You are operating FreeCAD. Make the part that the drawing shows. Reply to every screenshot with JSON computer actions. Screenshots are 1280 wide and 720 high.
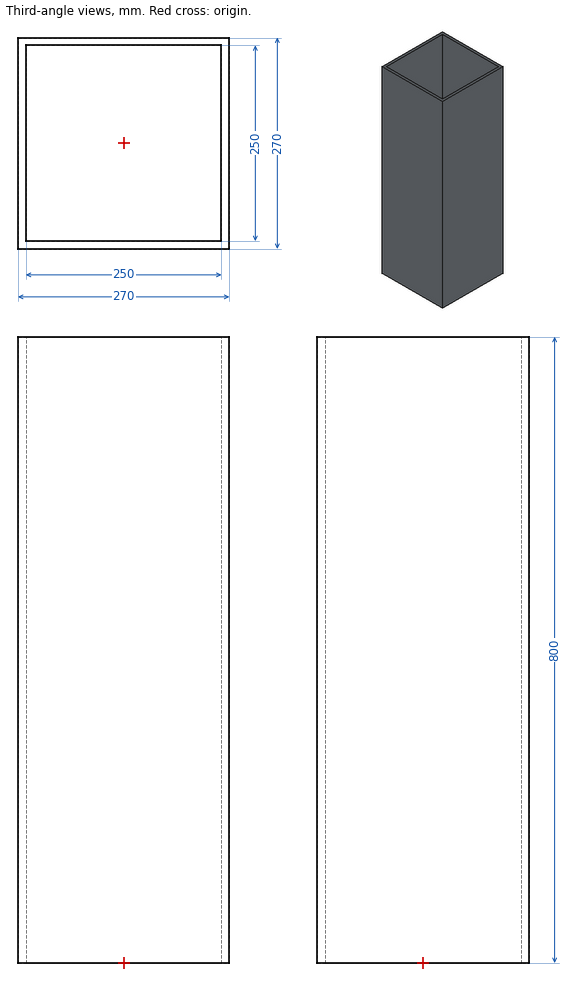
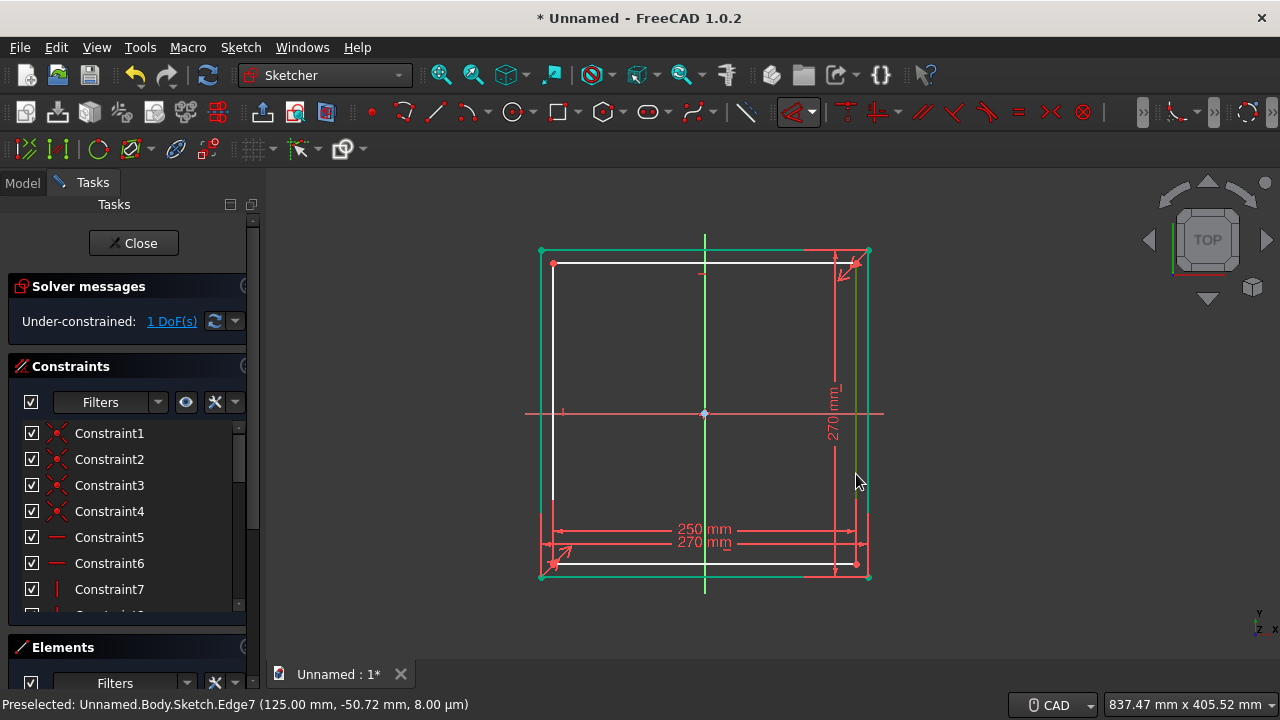
{"action": "left_click", "coordinate": [814, 112]}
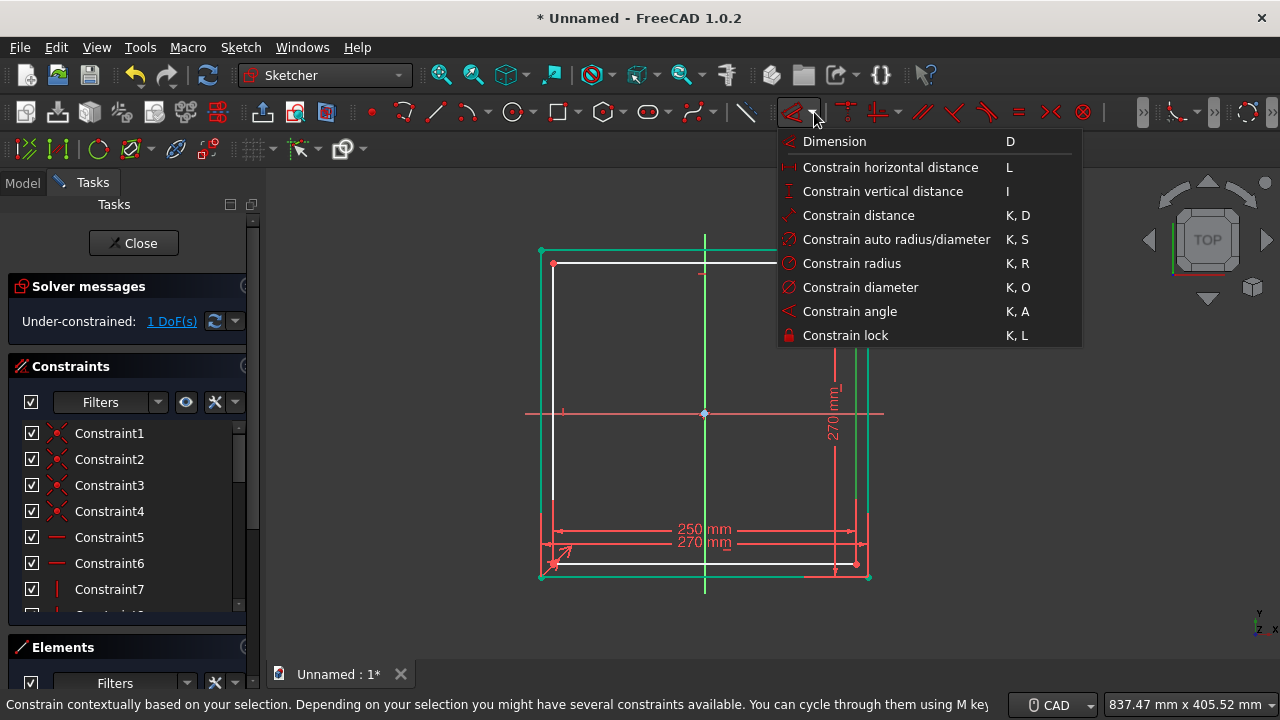
{"action": "left_click", "coordinate": [930, 191]}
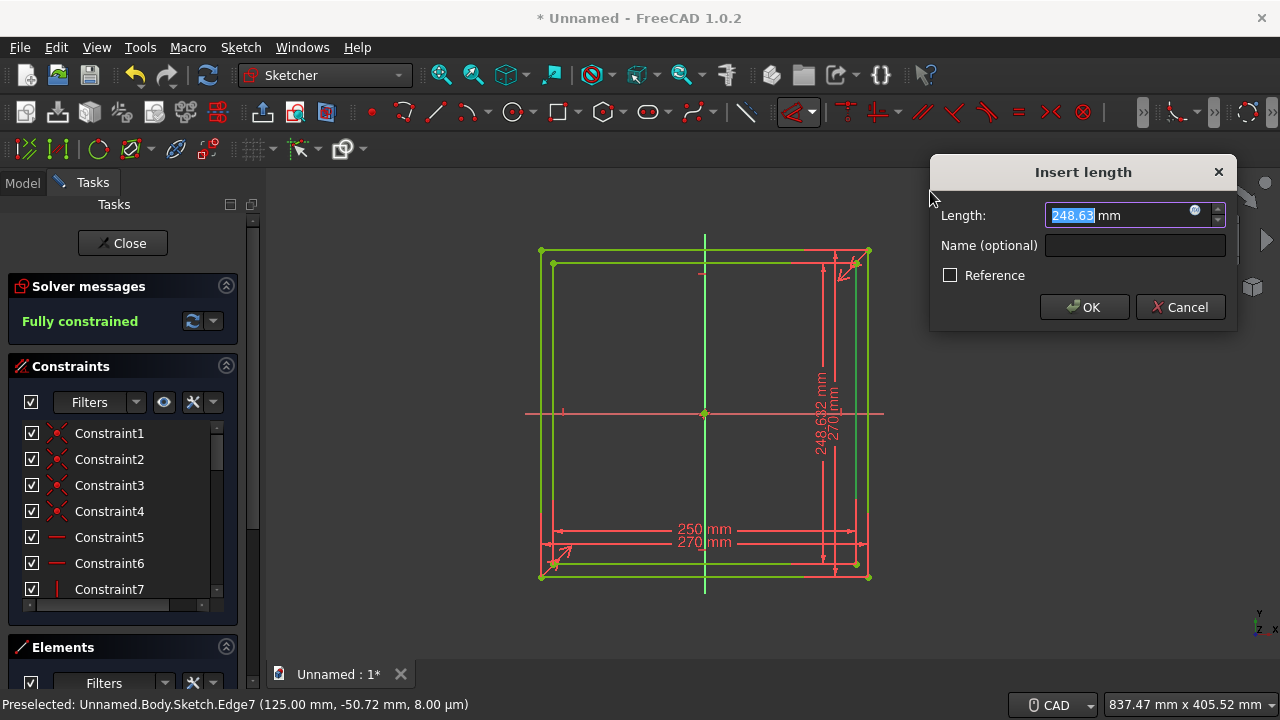
{"action": "type", "text": "250"}
{"action": "key", "text": "Return"}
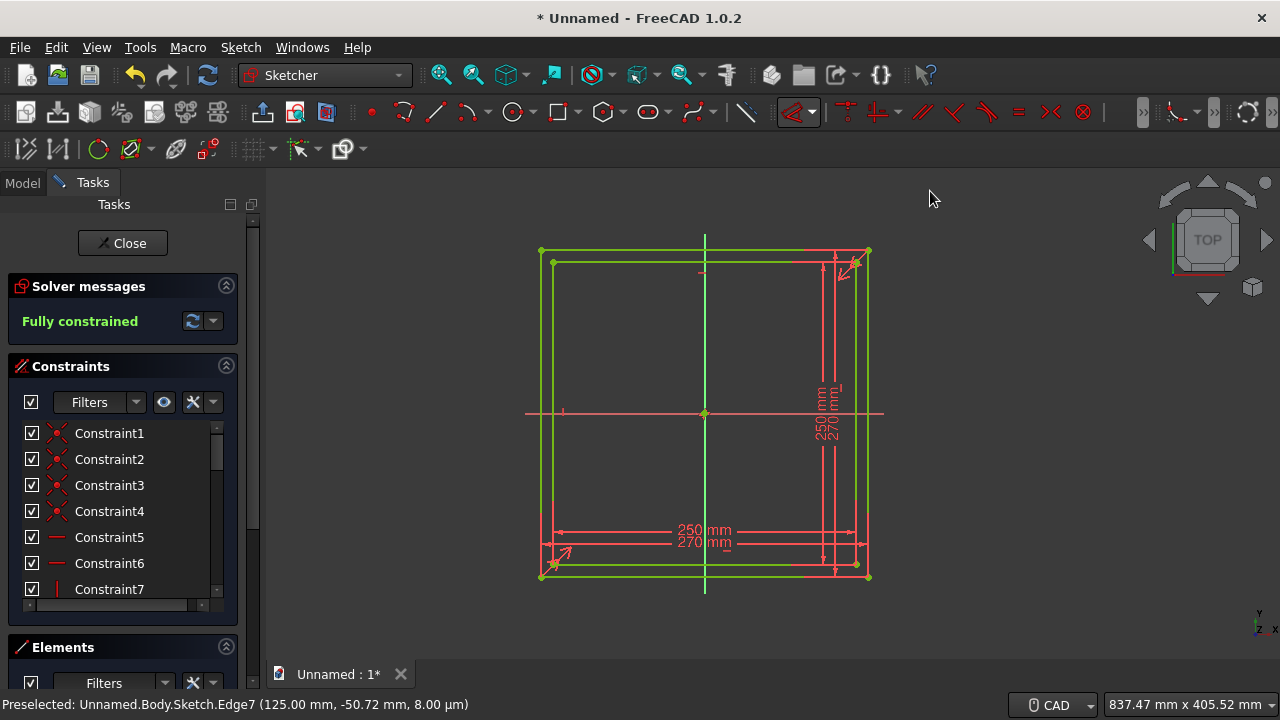
{"action": "left_click", "coordinate": [123, 243]}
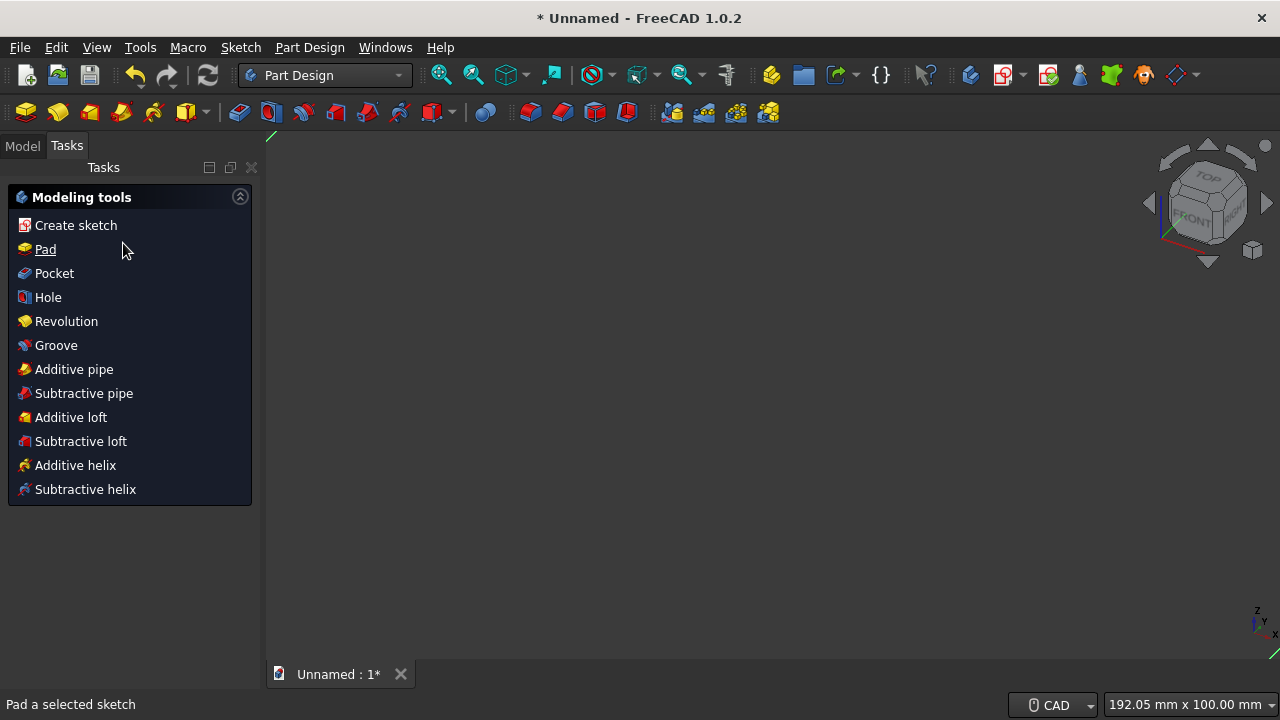
{"action": "left_click", "coordinate": [26, 112]}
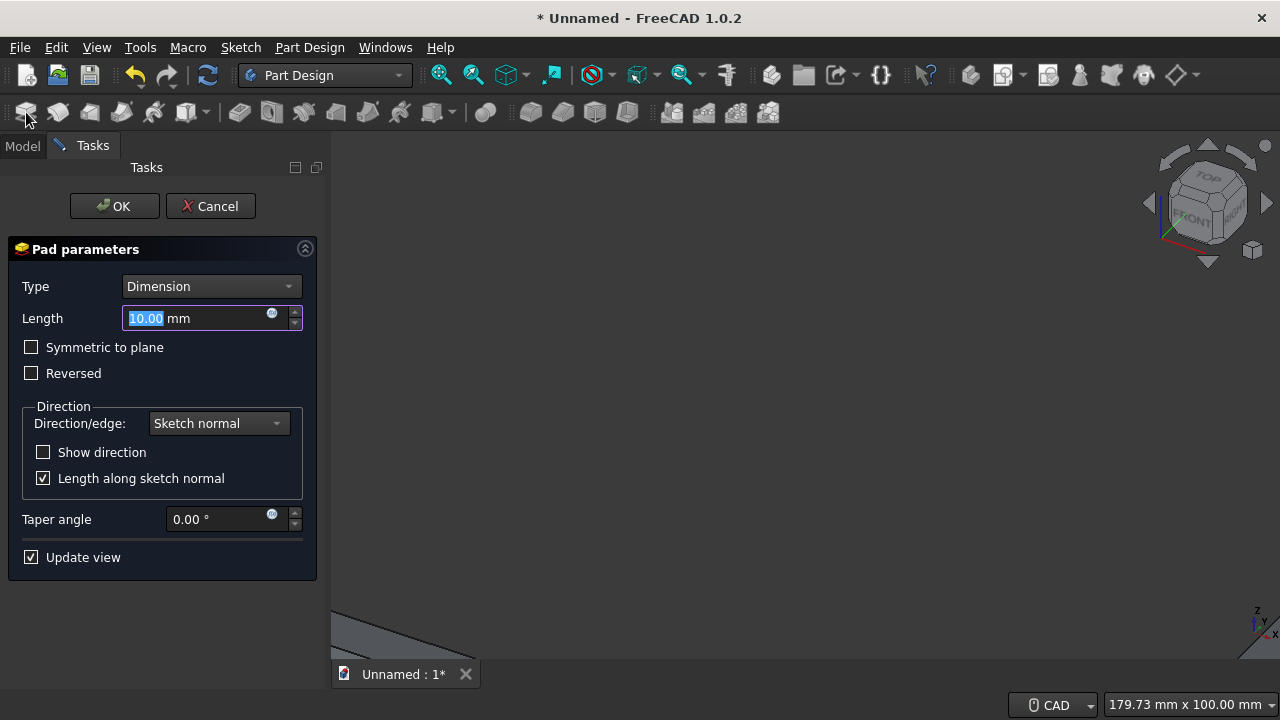
{"action": "type", "text": "800"}
{"action": "key", "text": "Tab"}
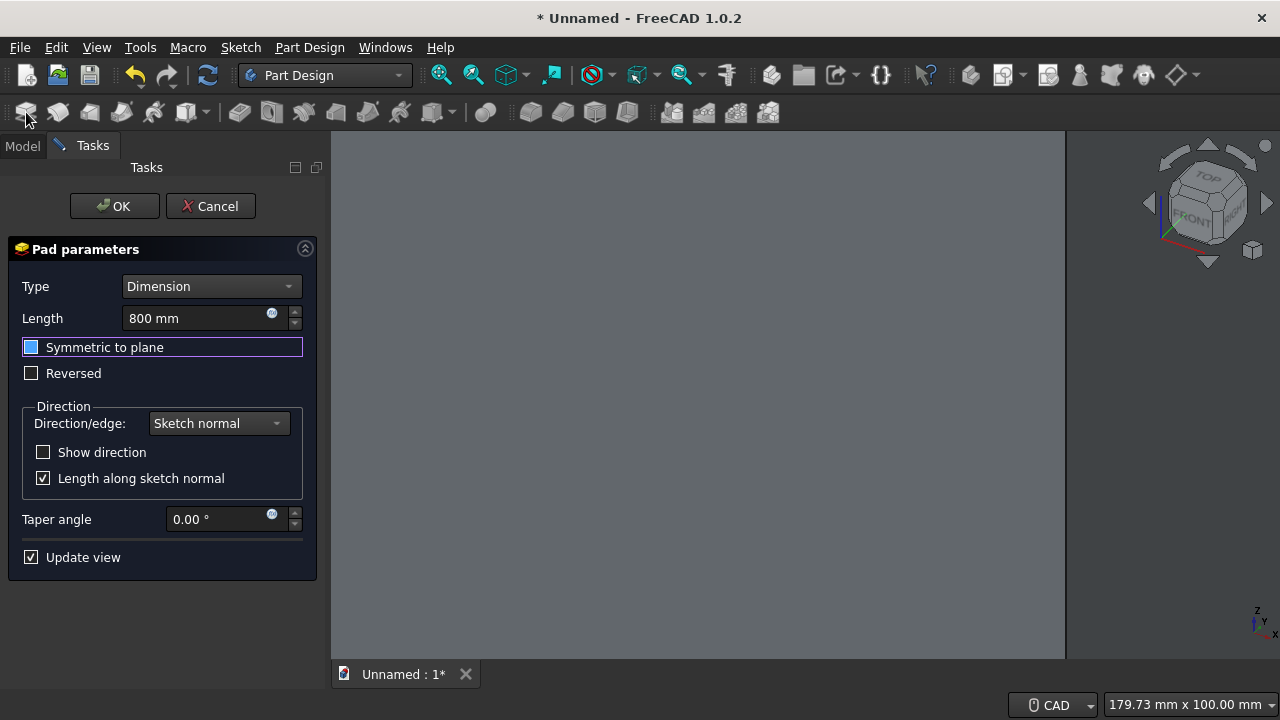
{"action": "left_click", "coordinate": [115, 206]}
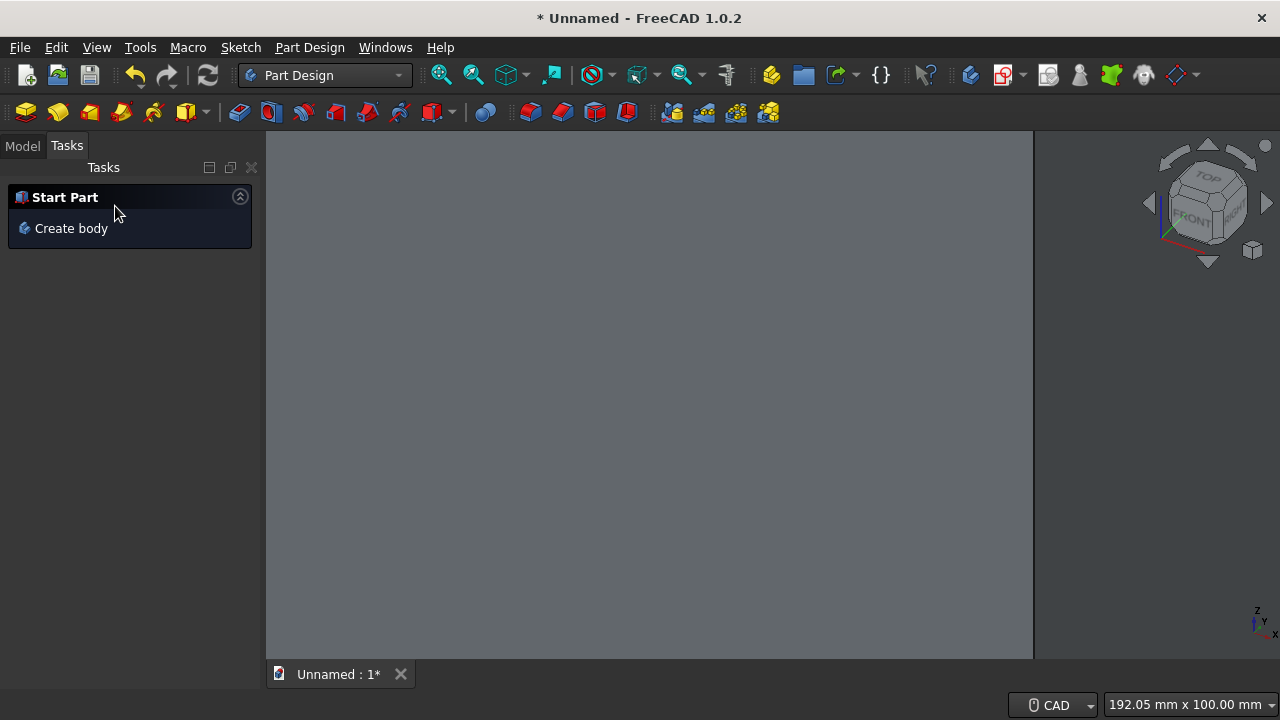
{"action": "key", "text": "0"}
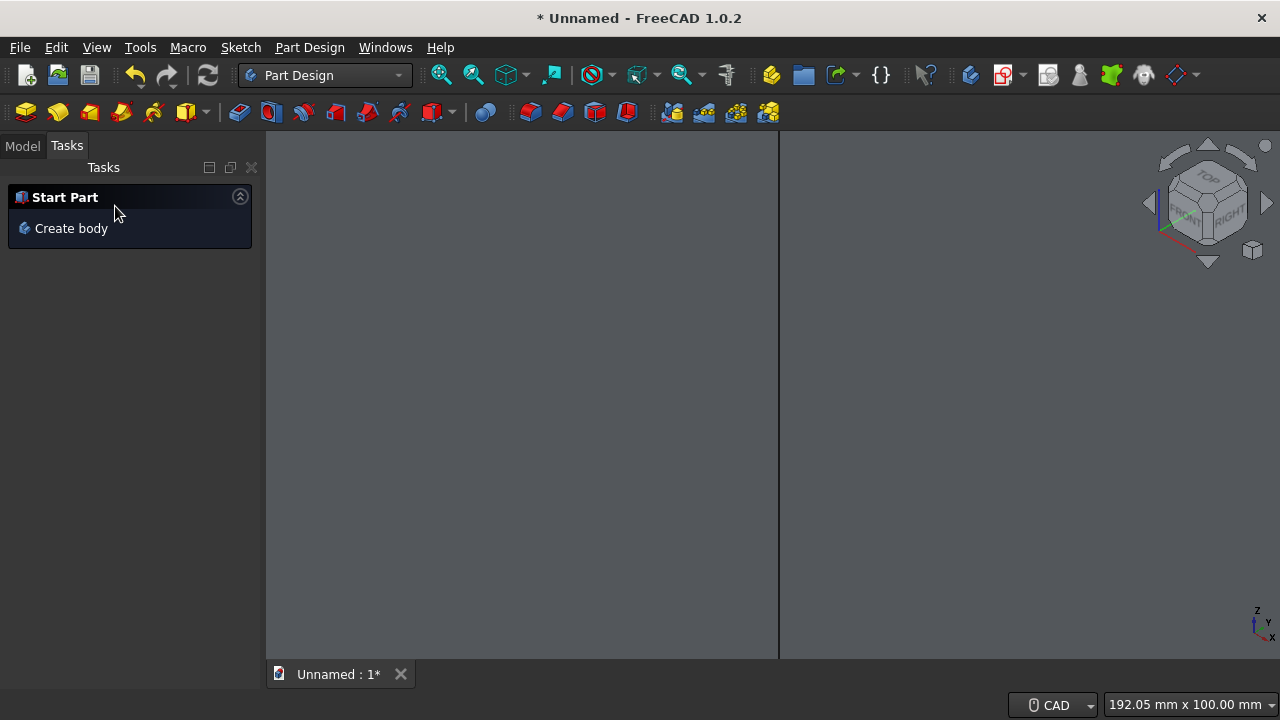
{"action": "key", "text": "v f"}